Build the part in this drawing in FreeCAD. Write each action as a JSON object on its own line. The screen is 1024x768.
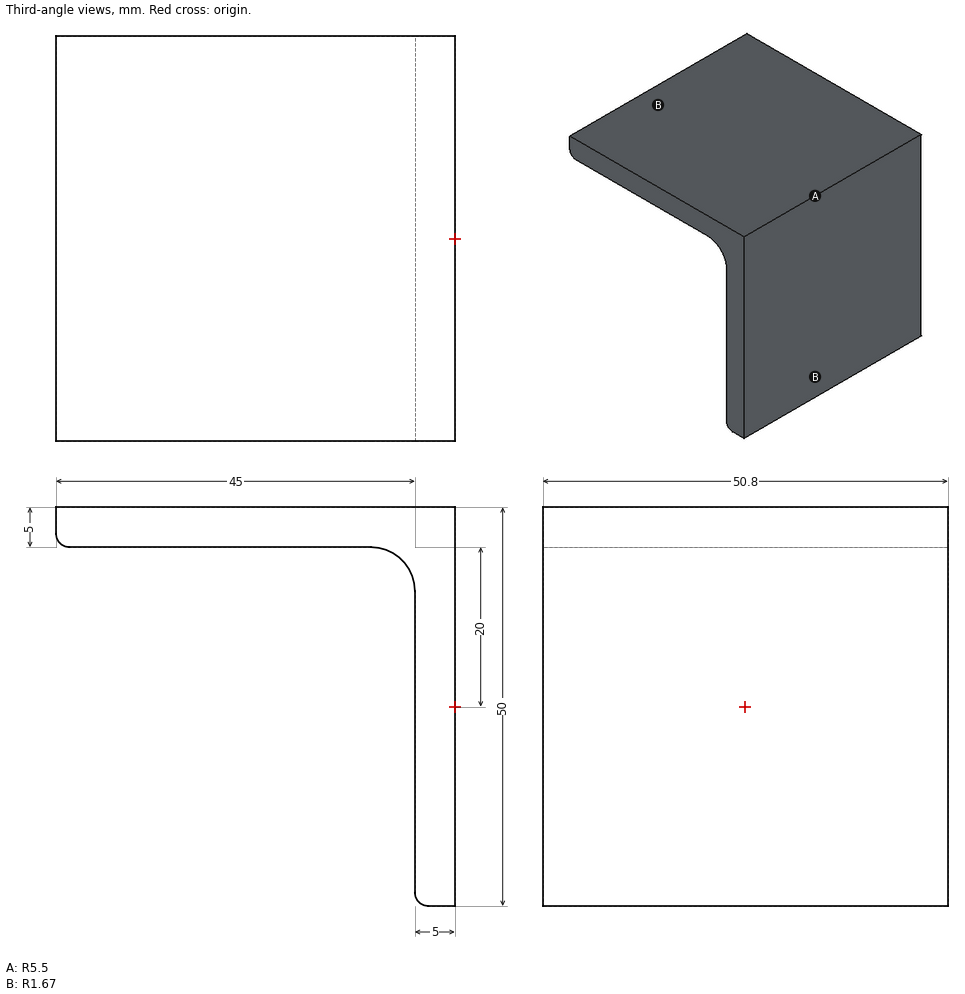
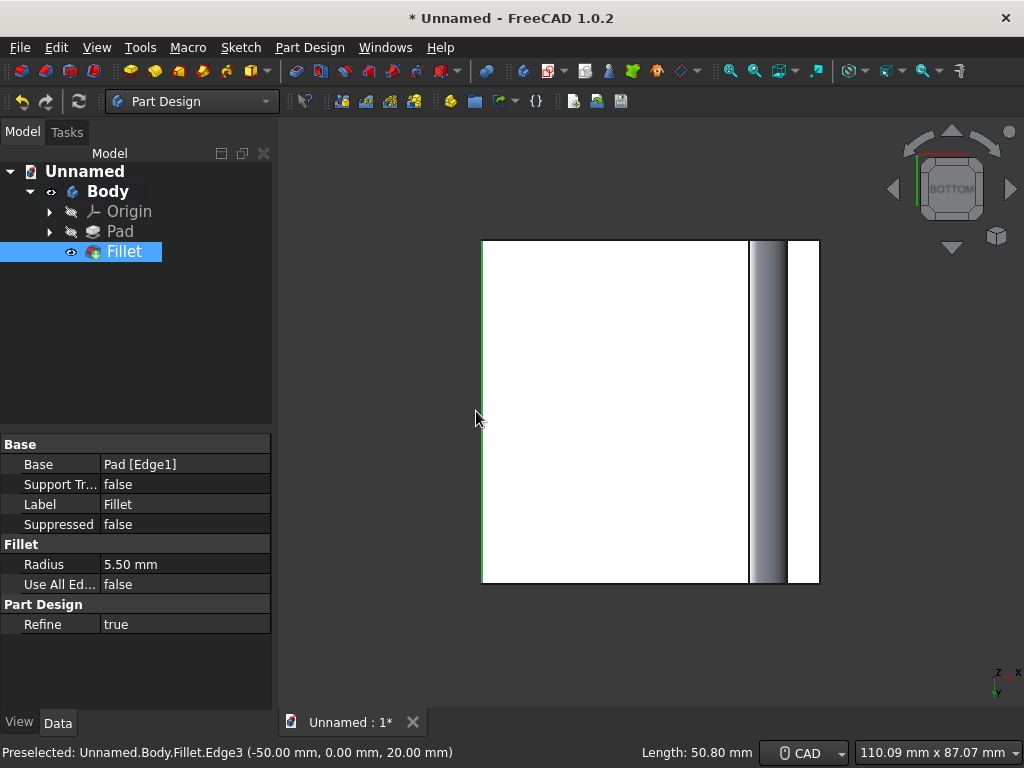
{"action": "left_click", "coordinate": [787, 411], "text": "ctrl"}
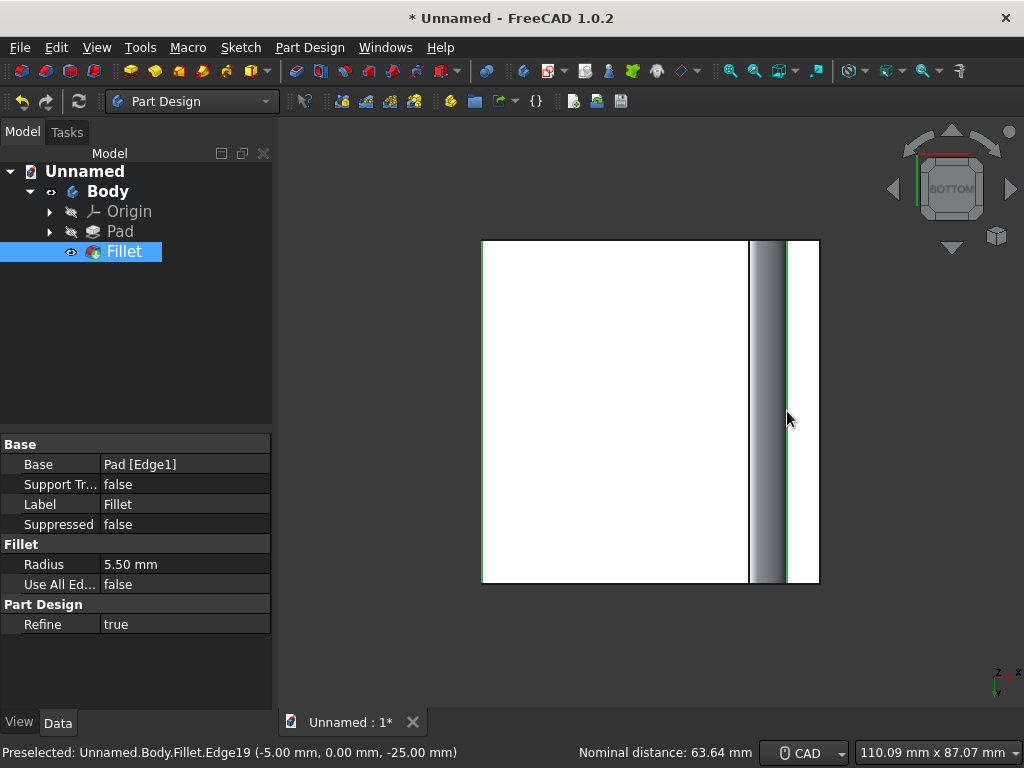
{"action": "left_click", "coordinate": [22, 72]}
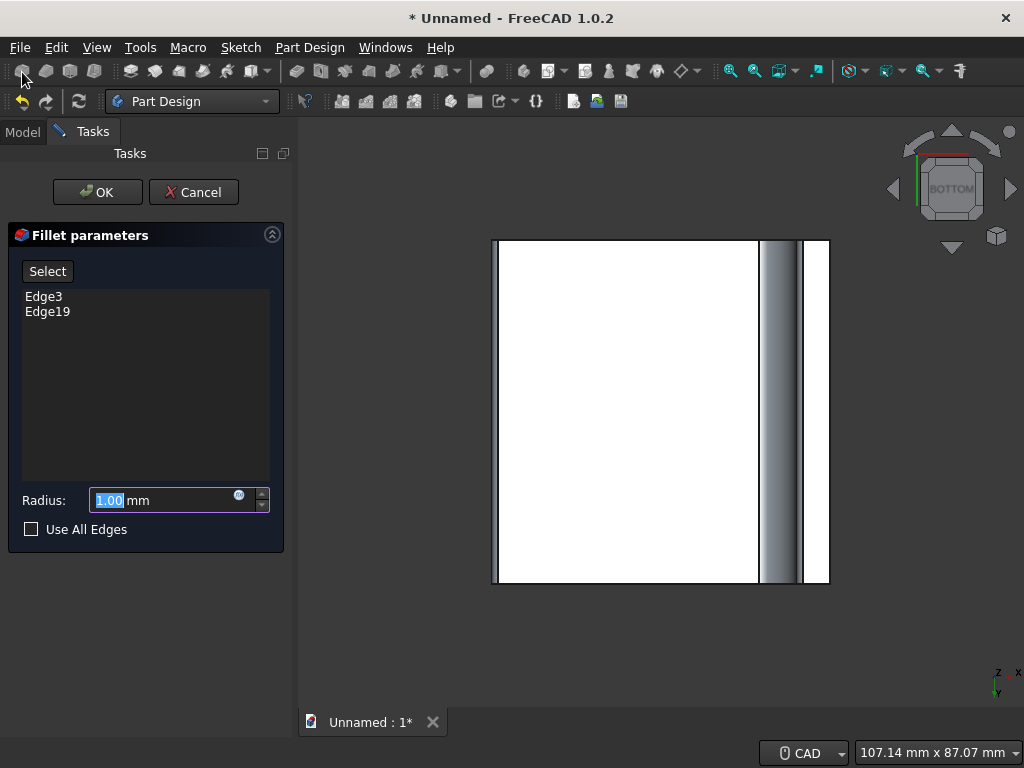
{"action": "type", "text": "1.67"}
{"action": "key", "text": "Tab"}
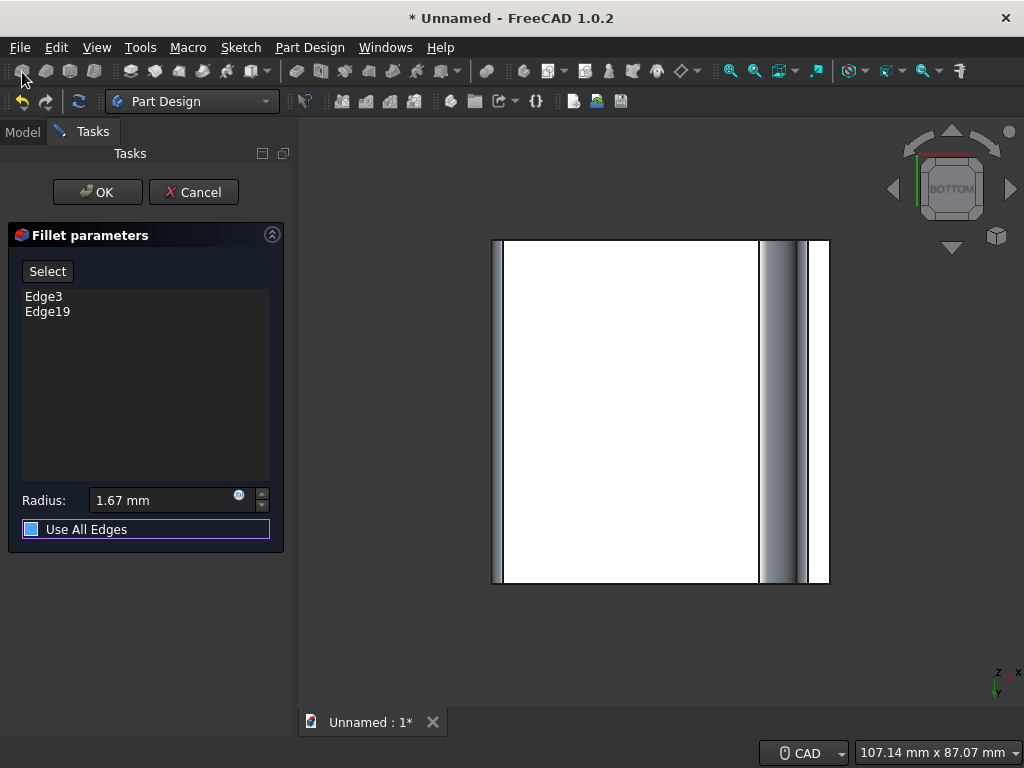
{"action": "left_click", "coordinate": [98, 192]}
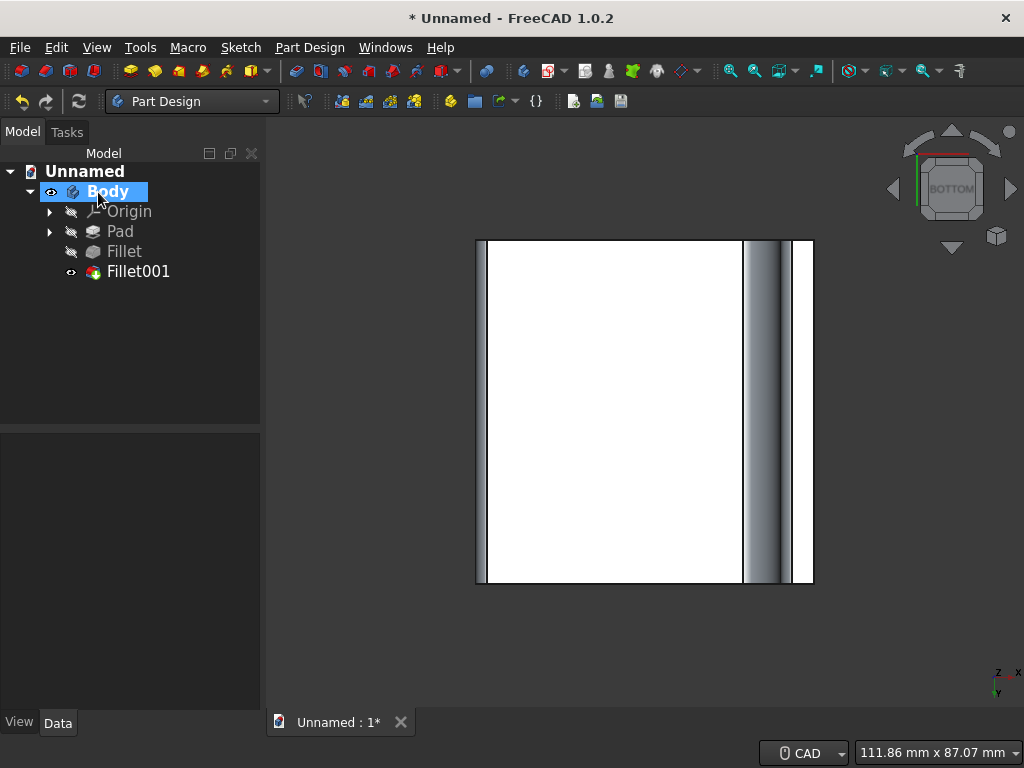
{"action": "key", "text": "0"}